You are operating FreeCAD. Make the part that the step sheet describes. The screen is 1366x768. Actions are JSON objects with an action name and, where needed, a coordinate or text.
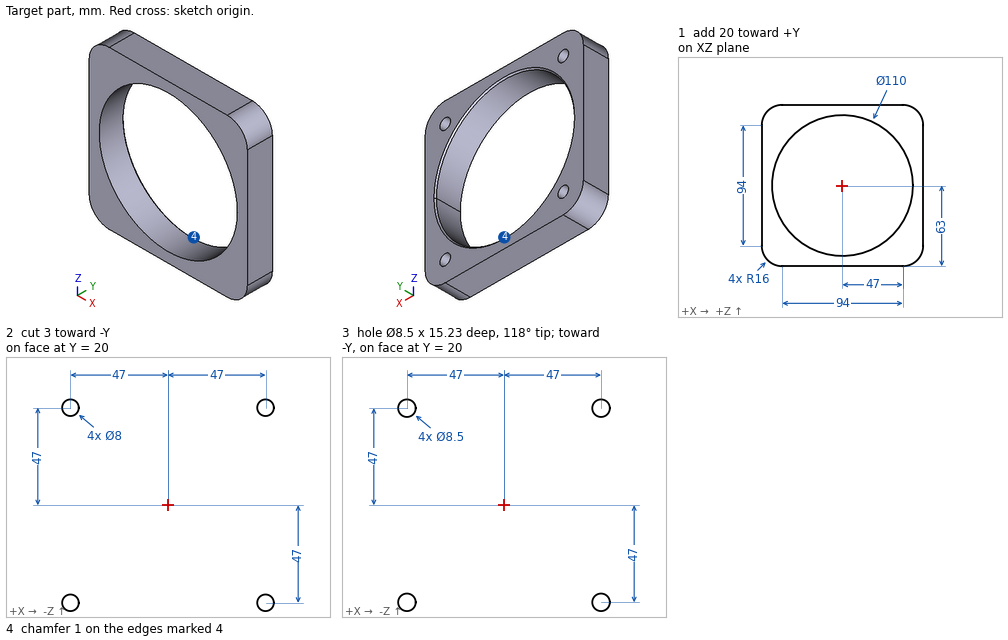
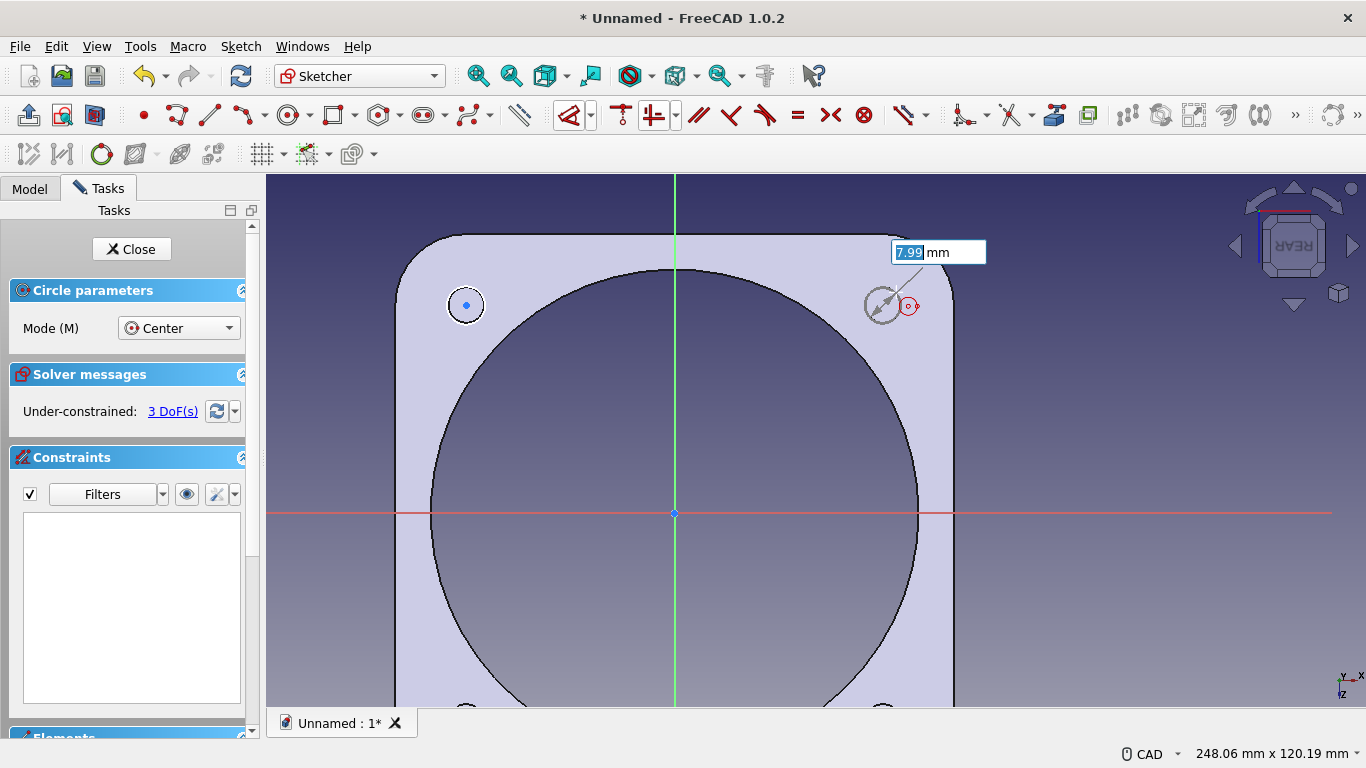
{"action": "left_click", "coordinate": [896, 292]}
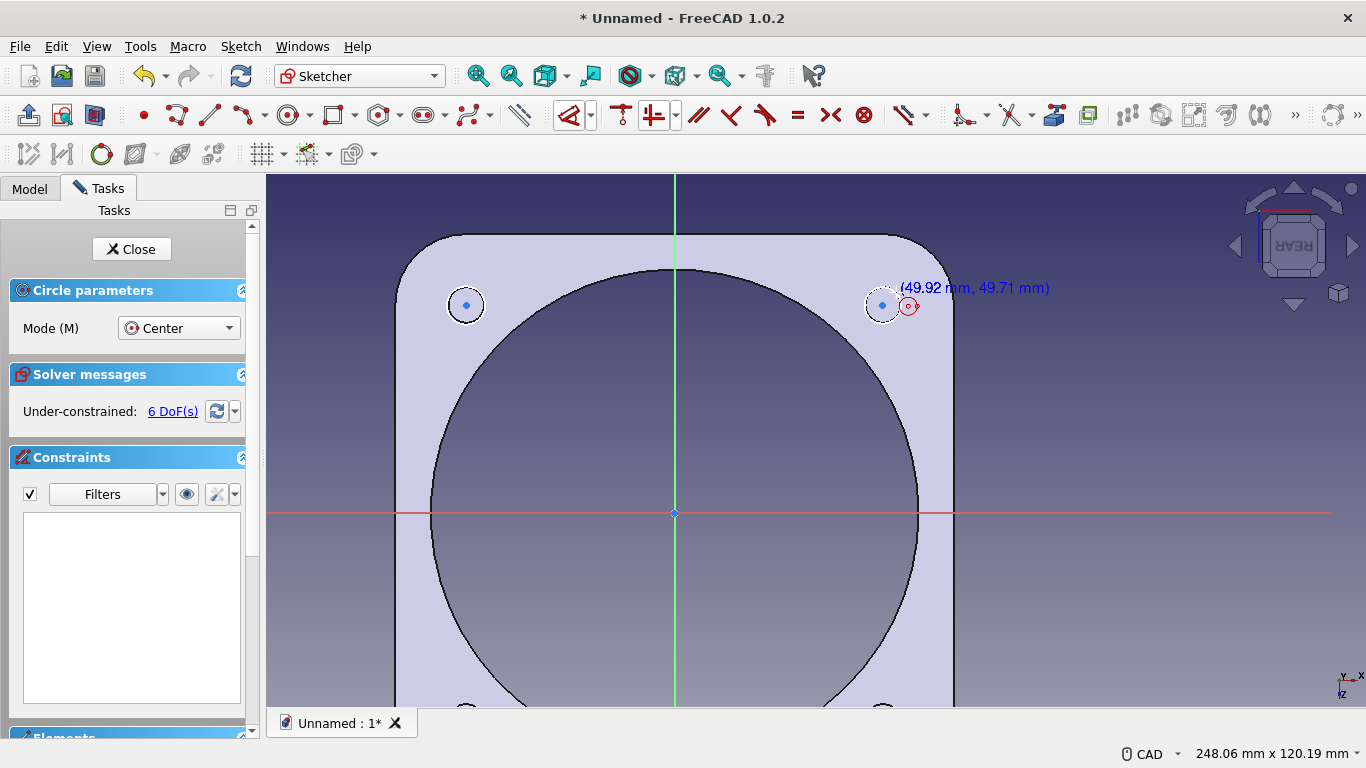
{"action": "scroll", "coordinate": [896, 292], "scroll_direction": "down", "scroll_amount": 2}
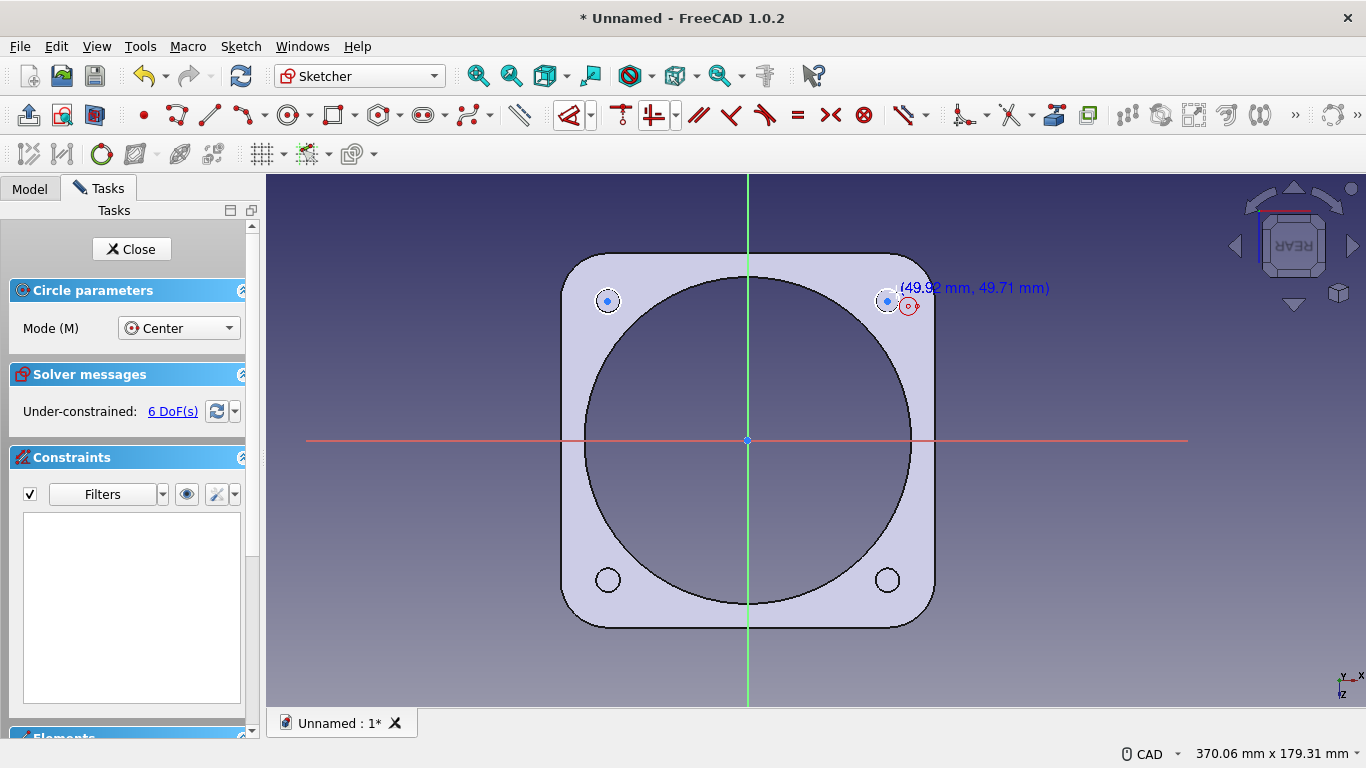
{"action": "scroll", "coordinate": [888, 580], "scroll_direction": "up", "scroll_amount": 3}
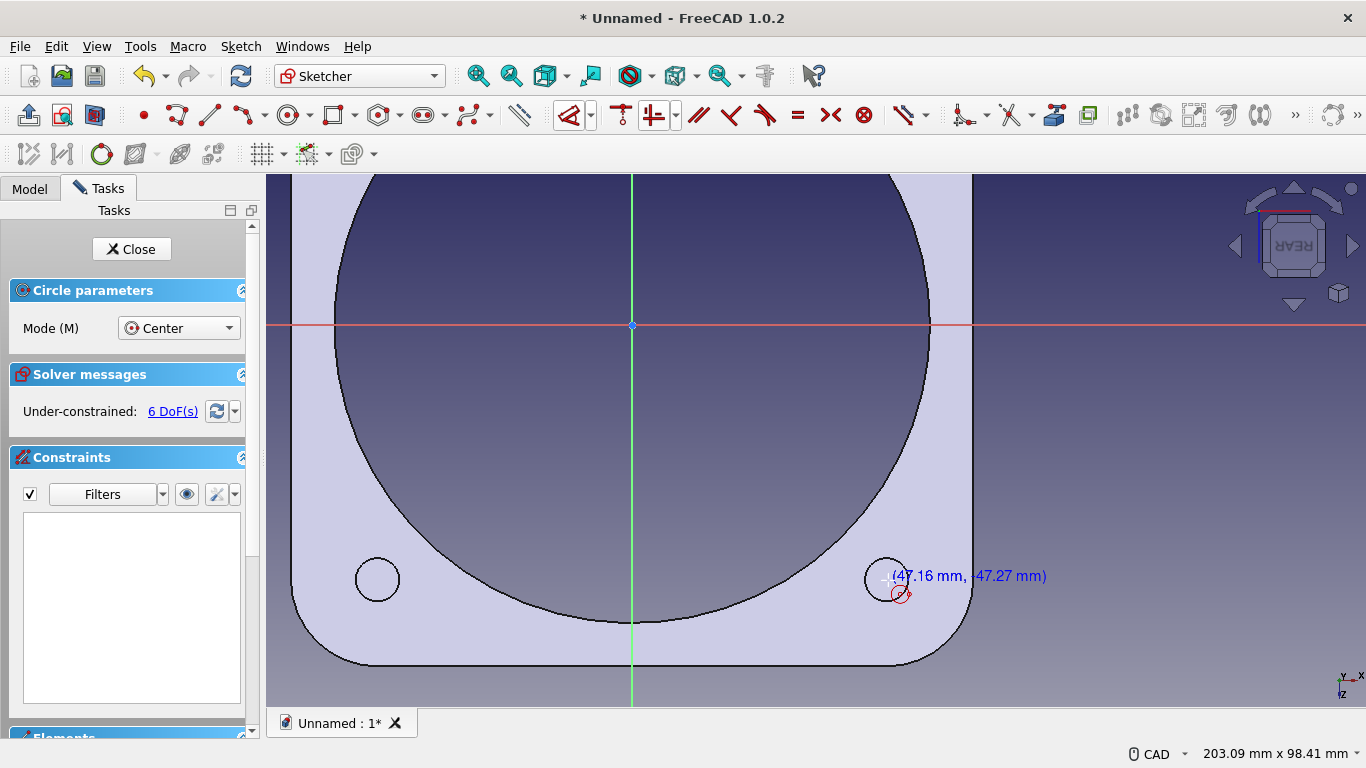
{"action": "left_click", "coordinate": [887, 580]}
{"action": "left_click", "coordinate": [903, 563]}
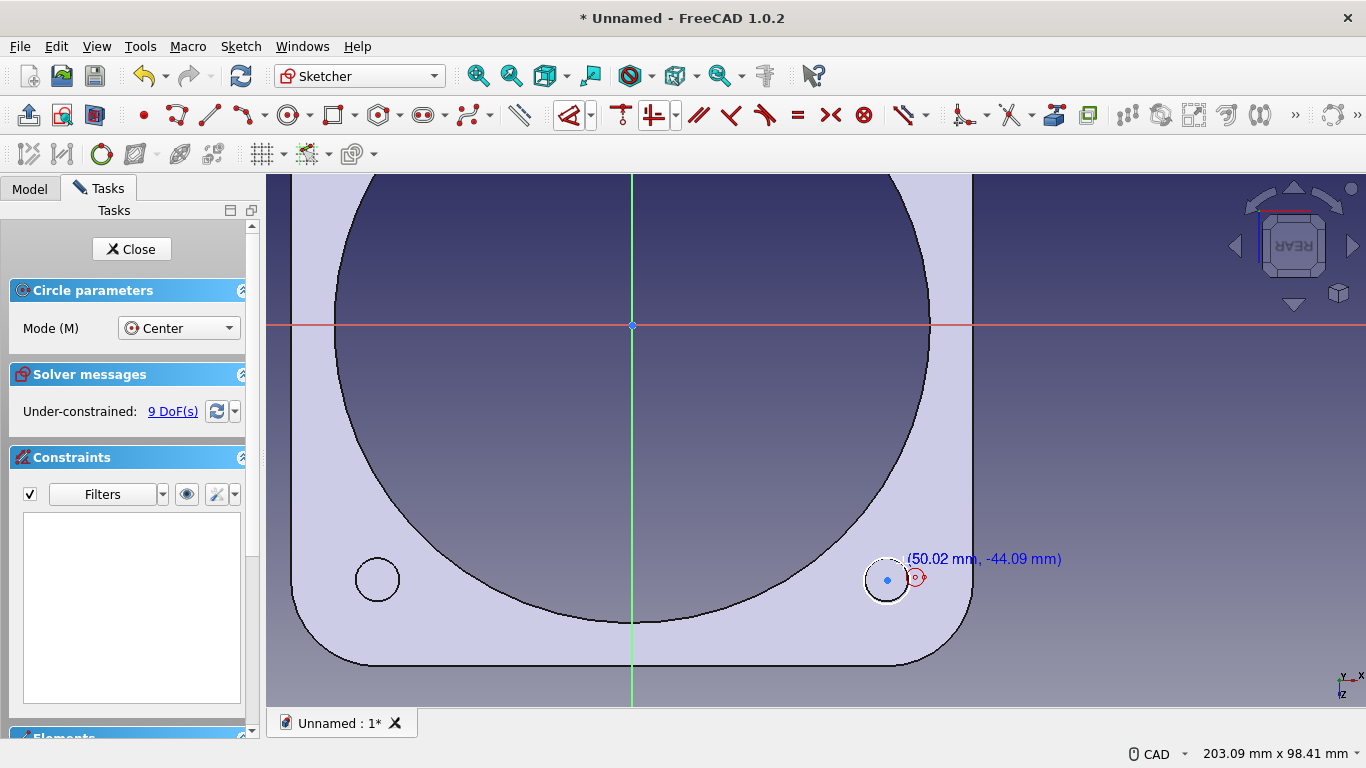
{"action": "left_click", "coordinate": [378, 580]}
{"action": "left_click", "coordinate": [394, 563]}
{"action": "key", "text": "Escape"}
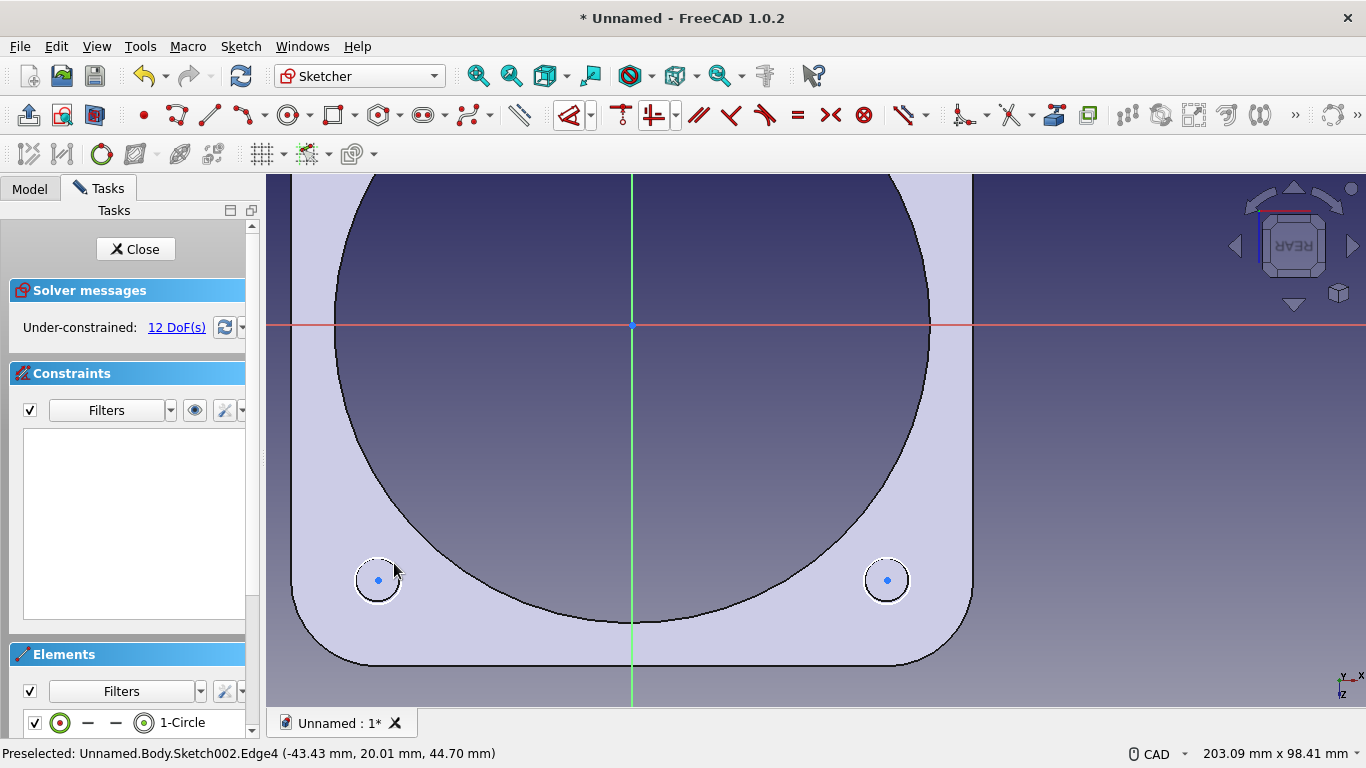
{"action": "scroll", "coordinate": [888, 581], "scroll_direction": "down", "scroll_amount": 3}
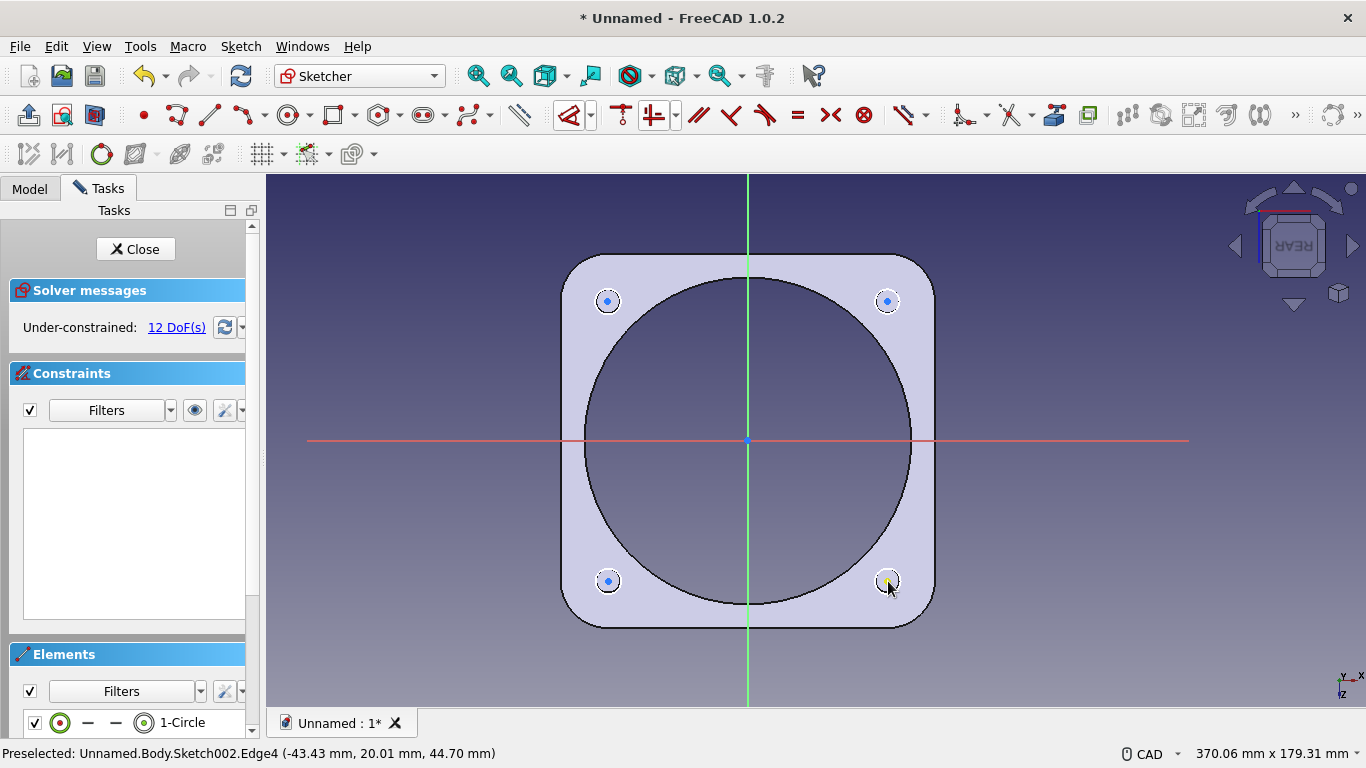
{"action": "left_click", "coordinate": [617, 292]}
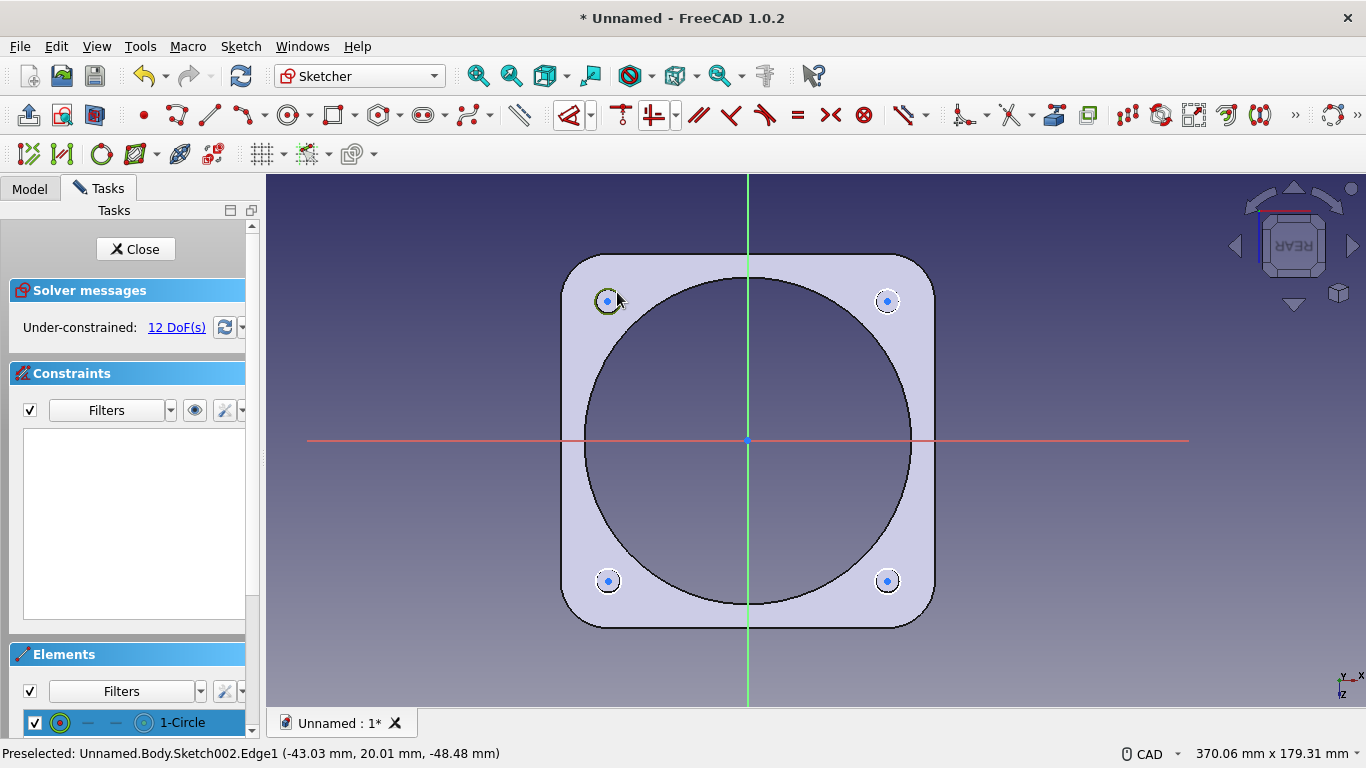
{"action": "left_click", "coordinate": [896, 293]}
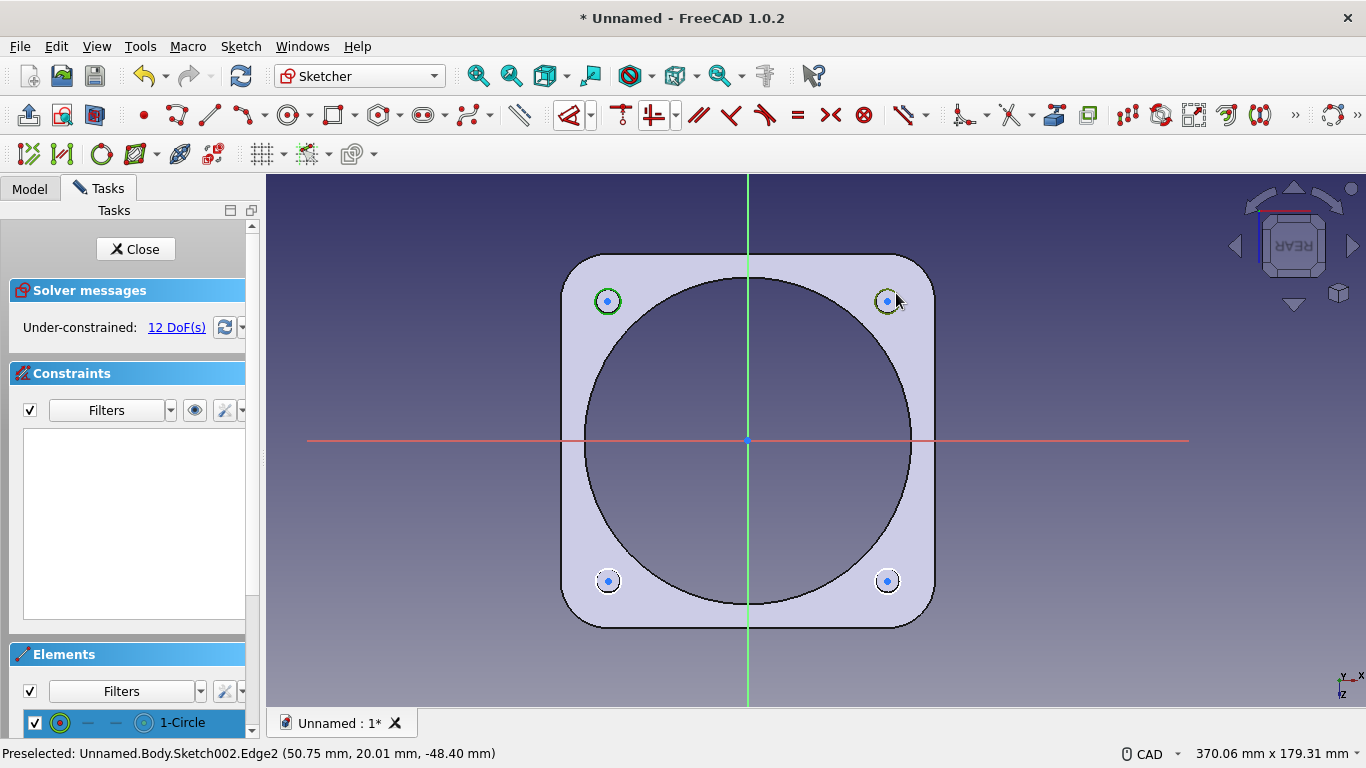
{"action": "left_click", "coordinate": [897, 572]}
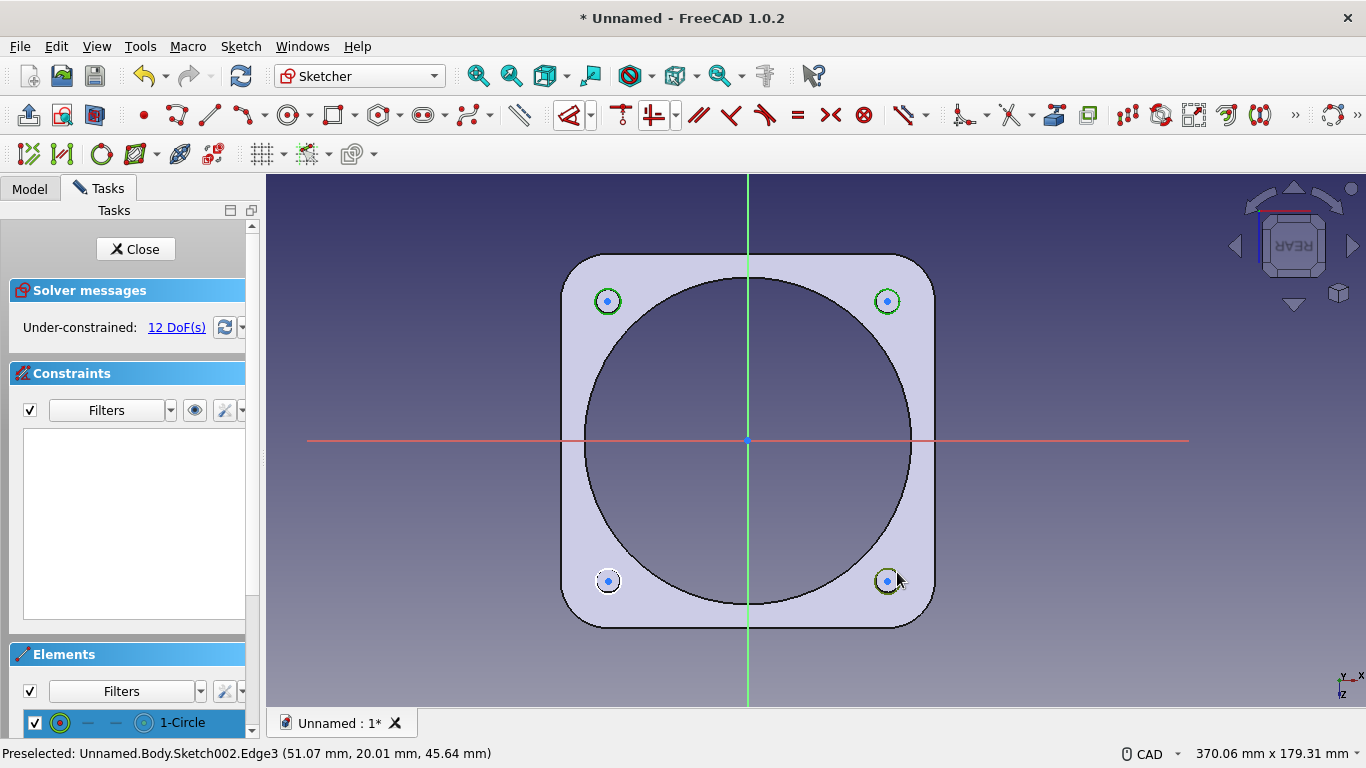
{"action": "left_click", "coordinate": [617, 572]}